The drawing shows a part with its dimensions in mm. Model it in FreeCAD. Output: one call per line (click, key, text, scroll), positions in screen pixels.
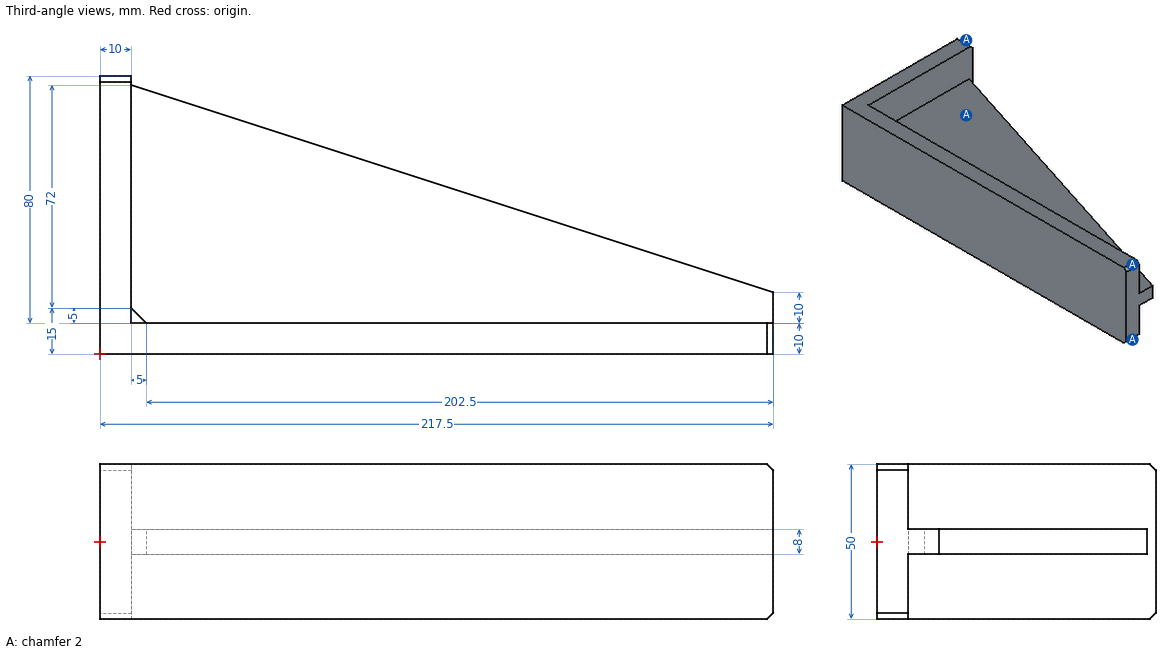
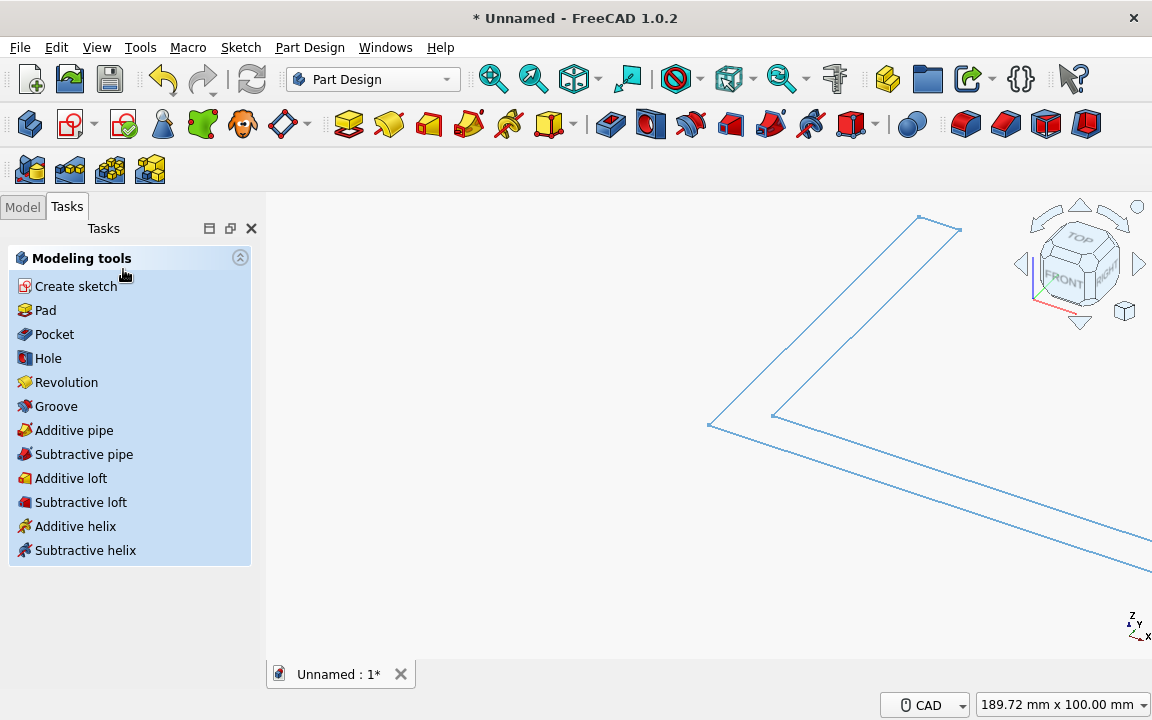
click(350, 124)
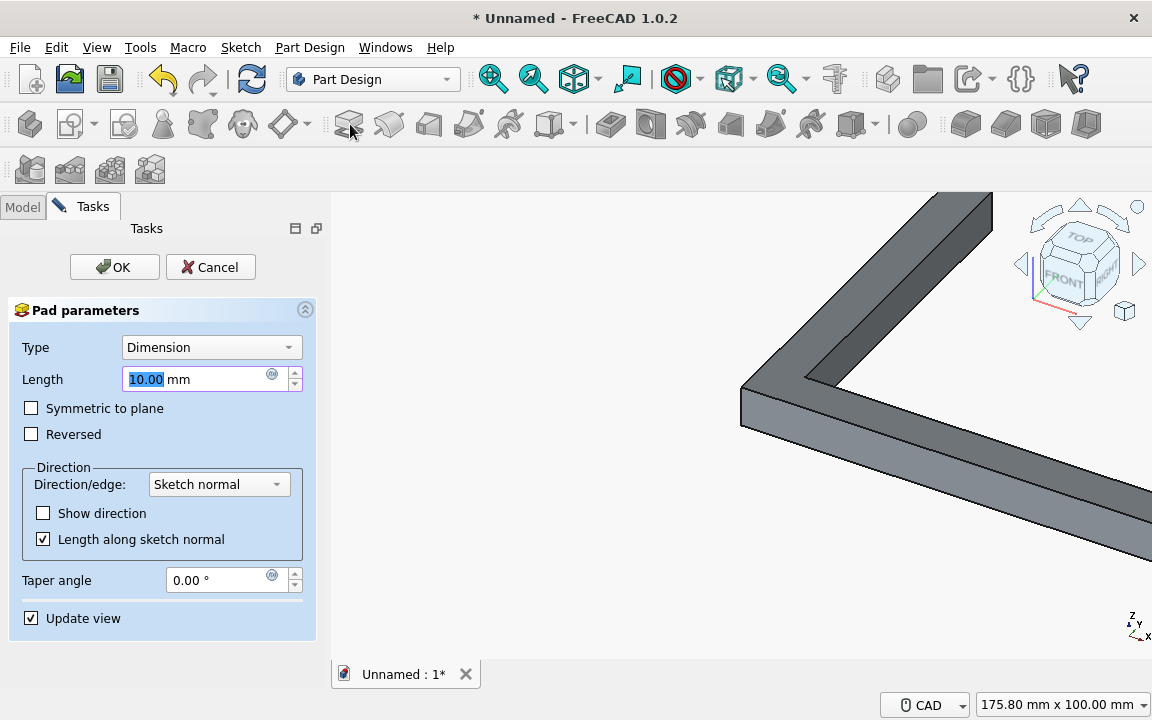
text(50)
key(Tab)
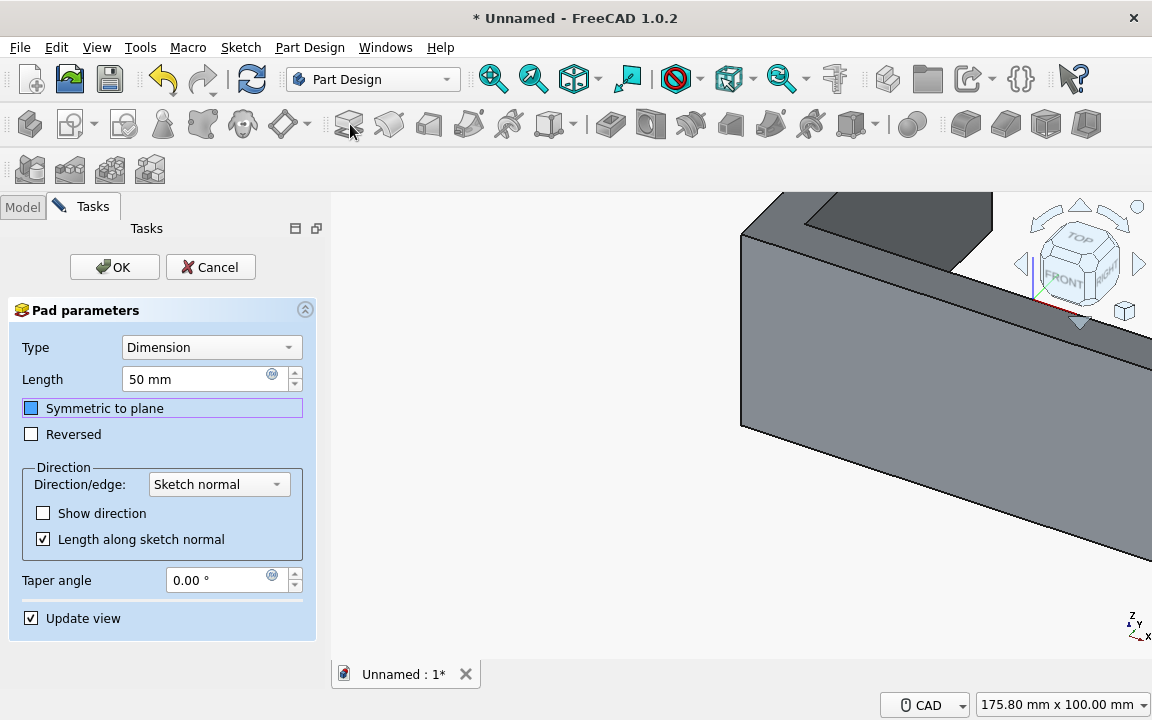
click(30, 408)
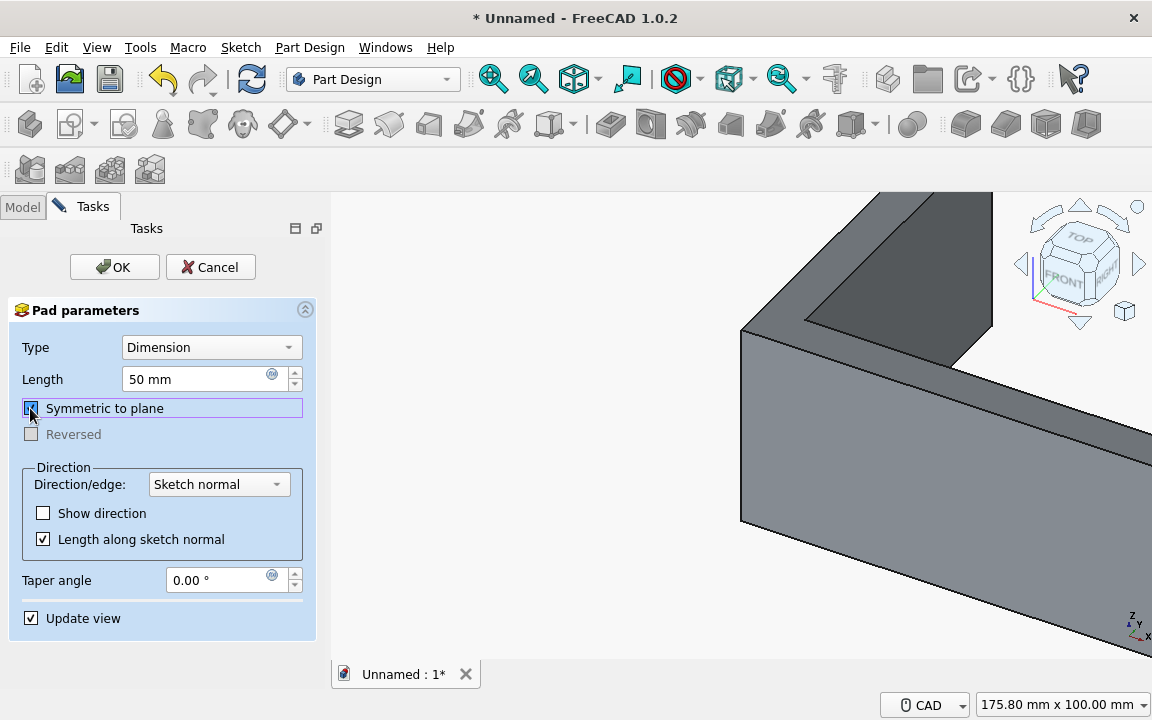
click(115, 267)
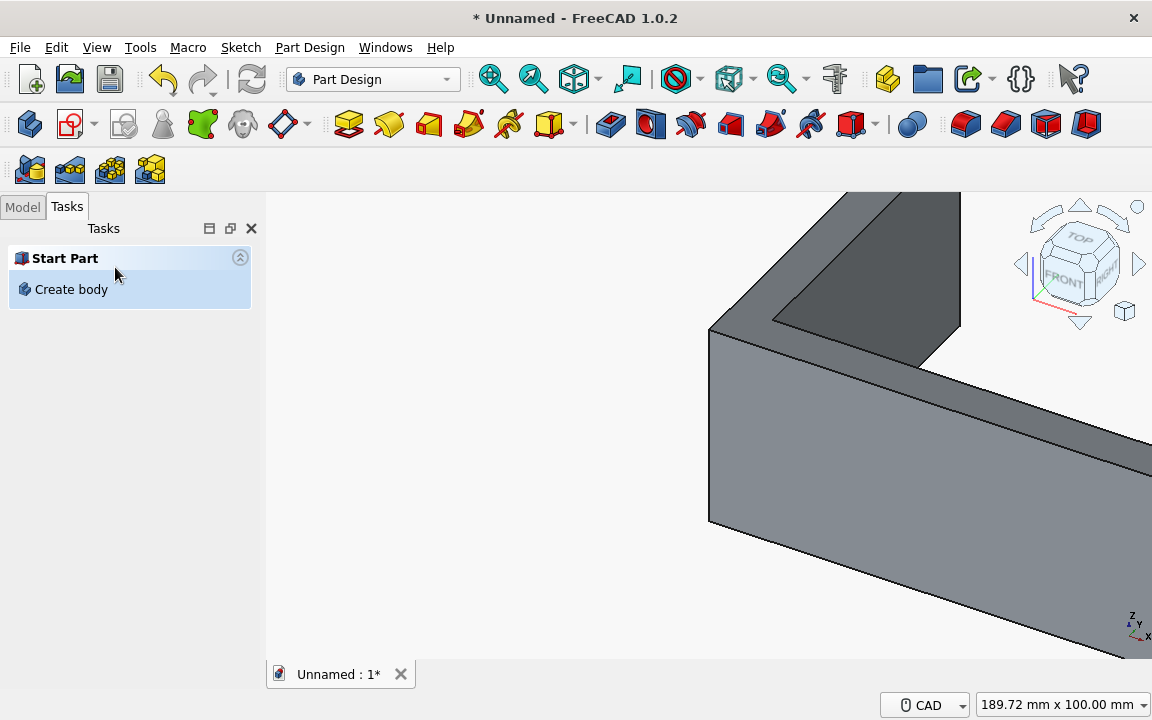
click(494, 80)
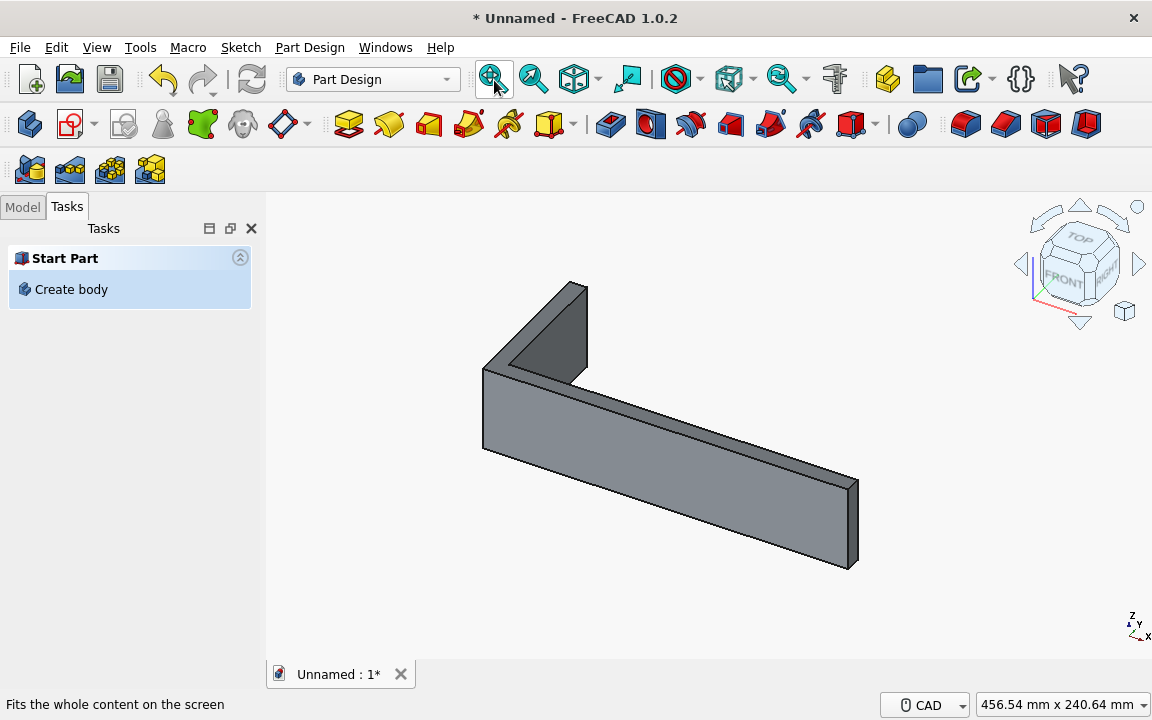
click(70, 124)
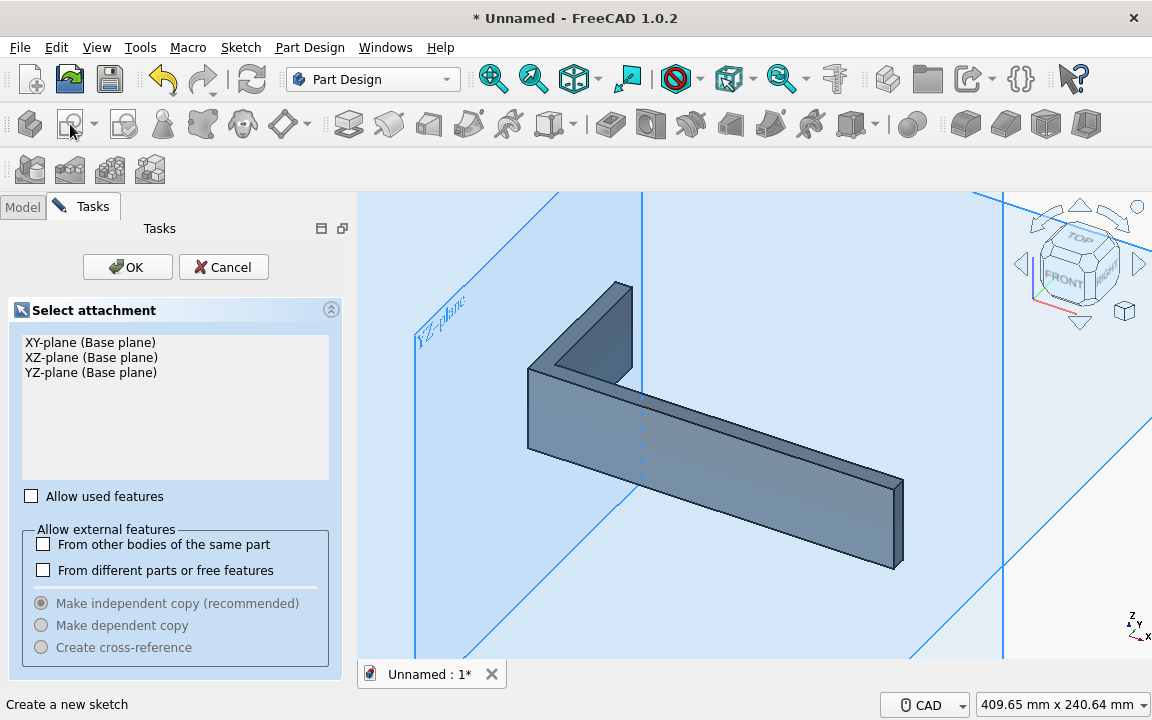
click(82, 342)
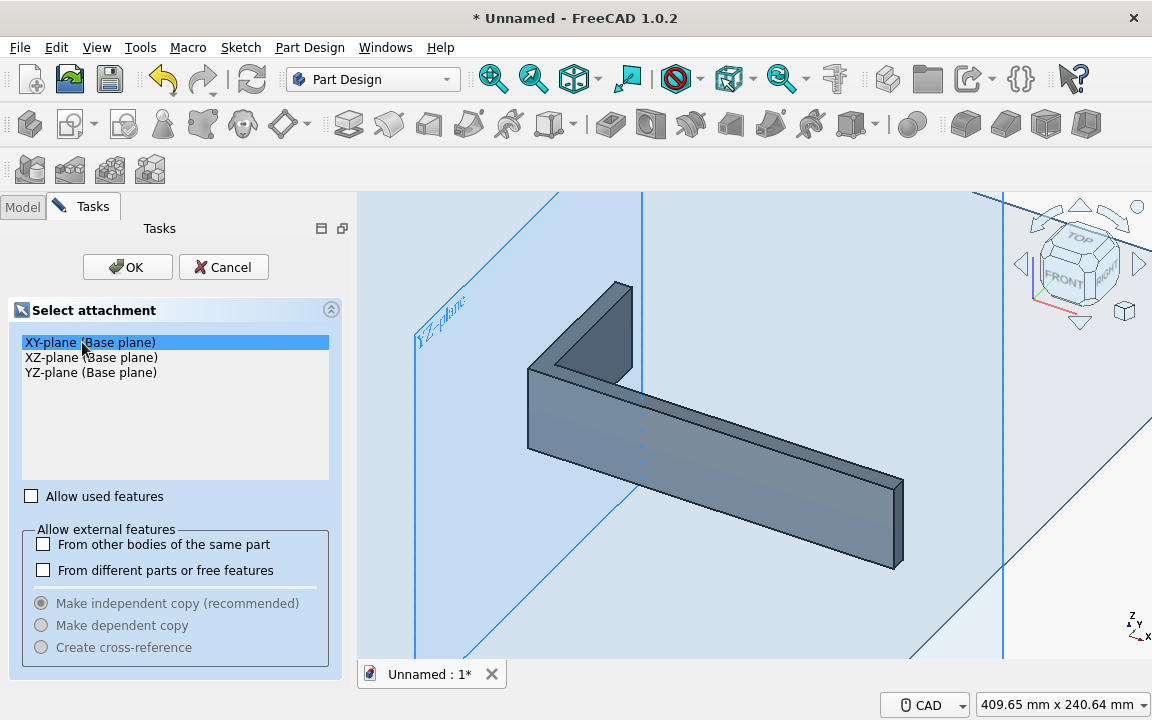
click(128, 267)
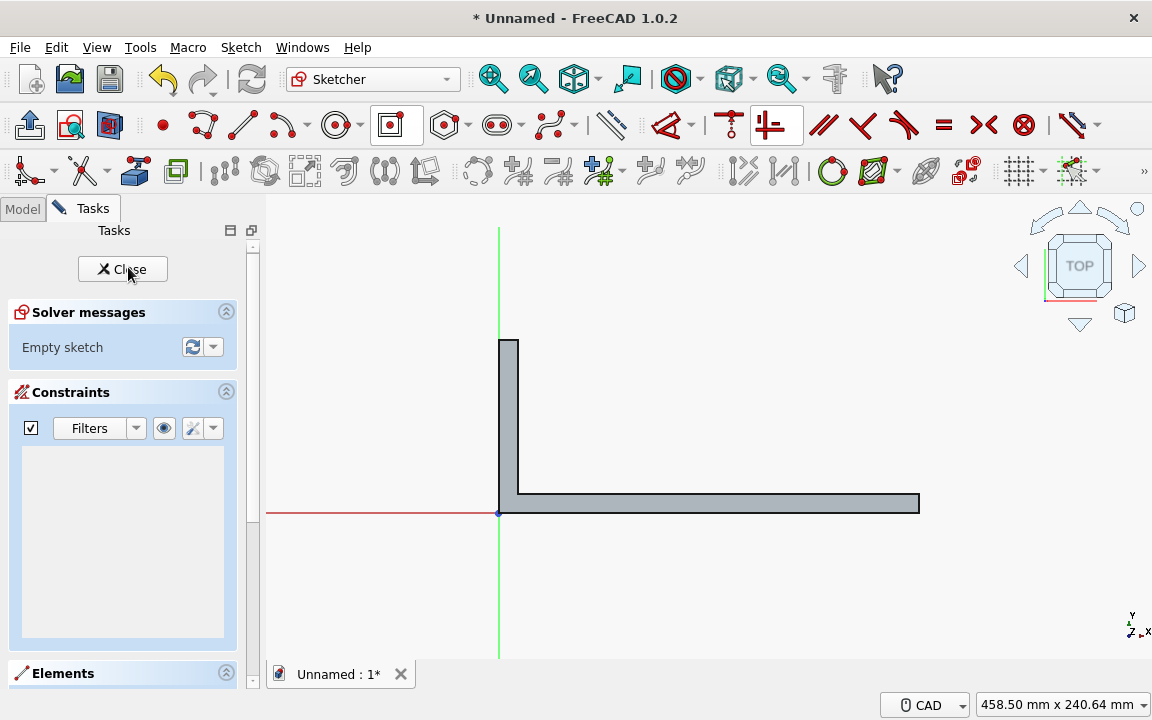
click(110, 126)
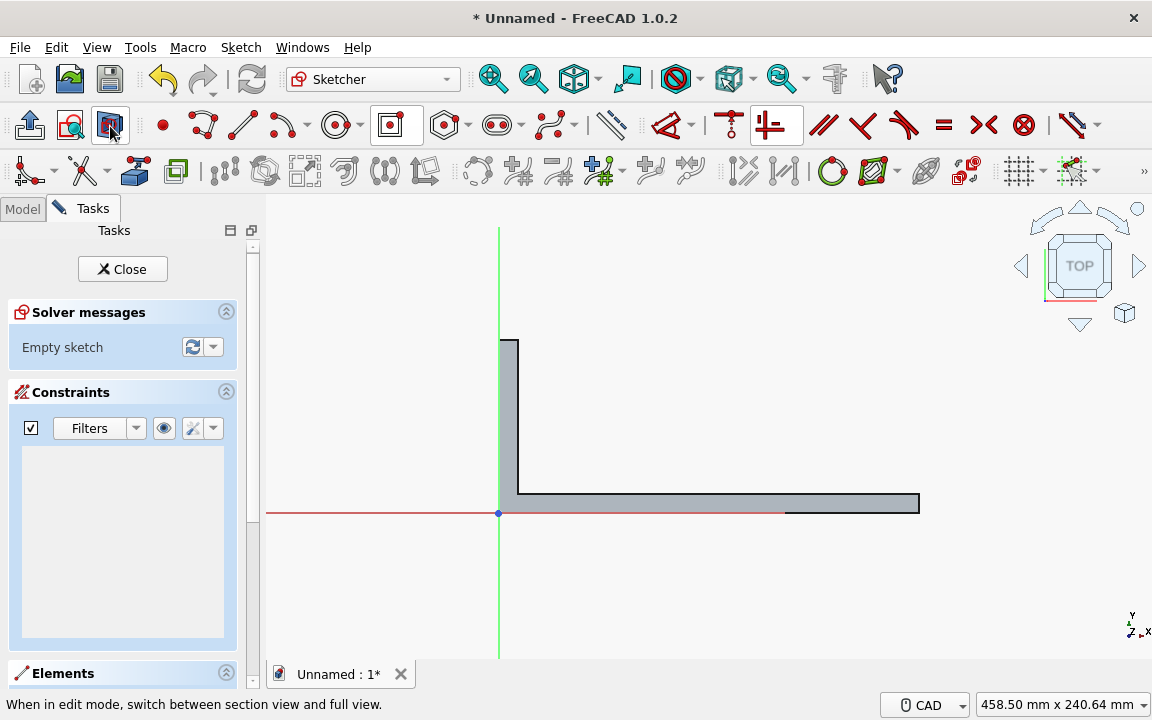
click(204, 126)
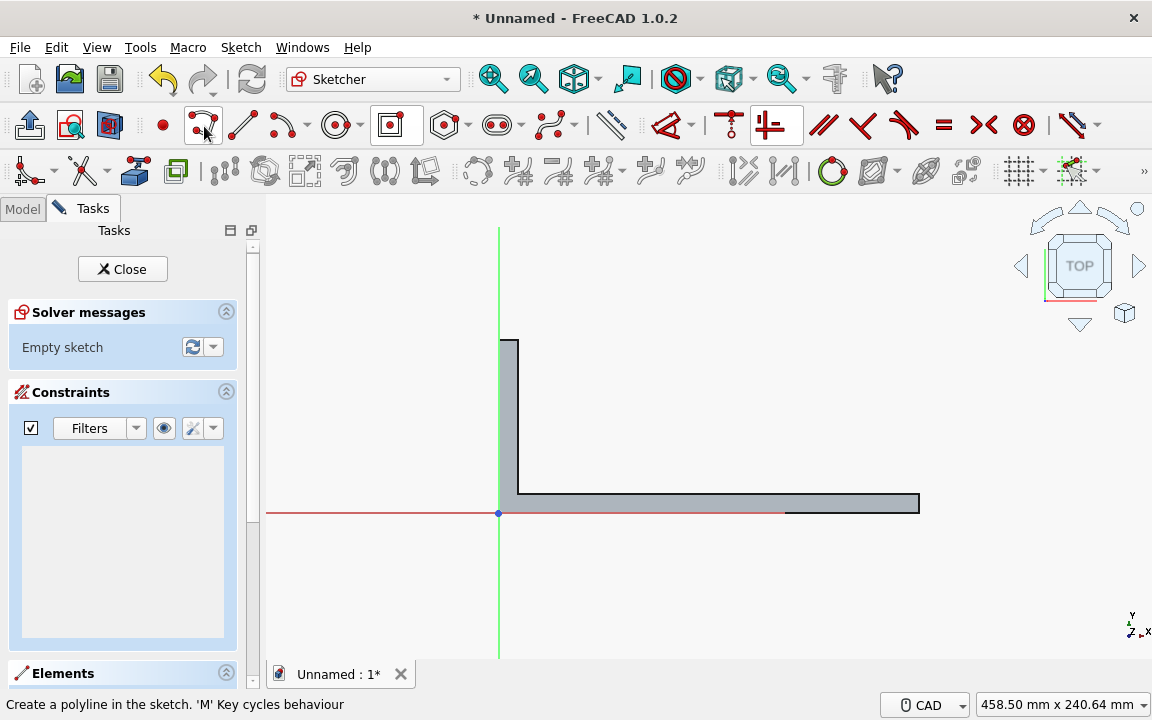
click(518, 484)
click(528, 494)
click(919, 494)
click(919, 475)
click(518, 345)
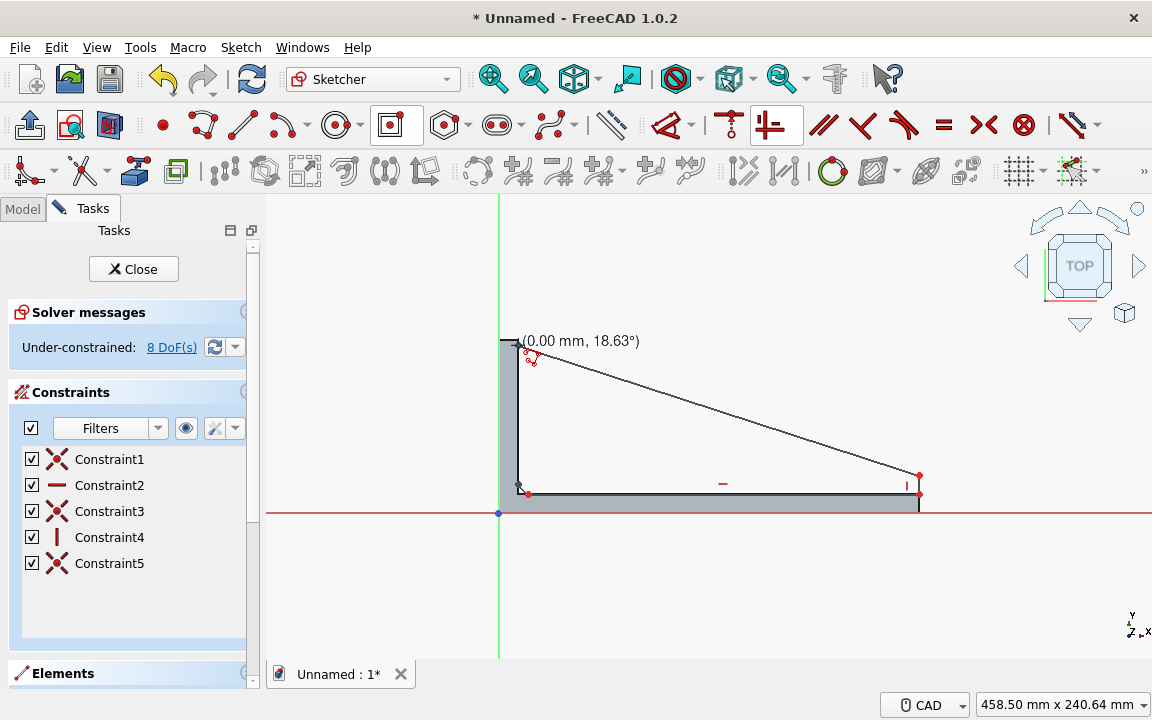
scroll(518, 484, up, 5)